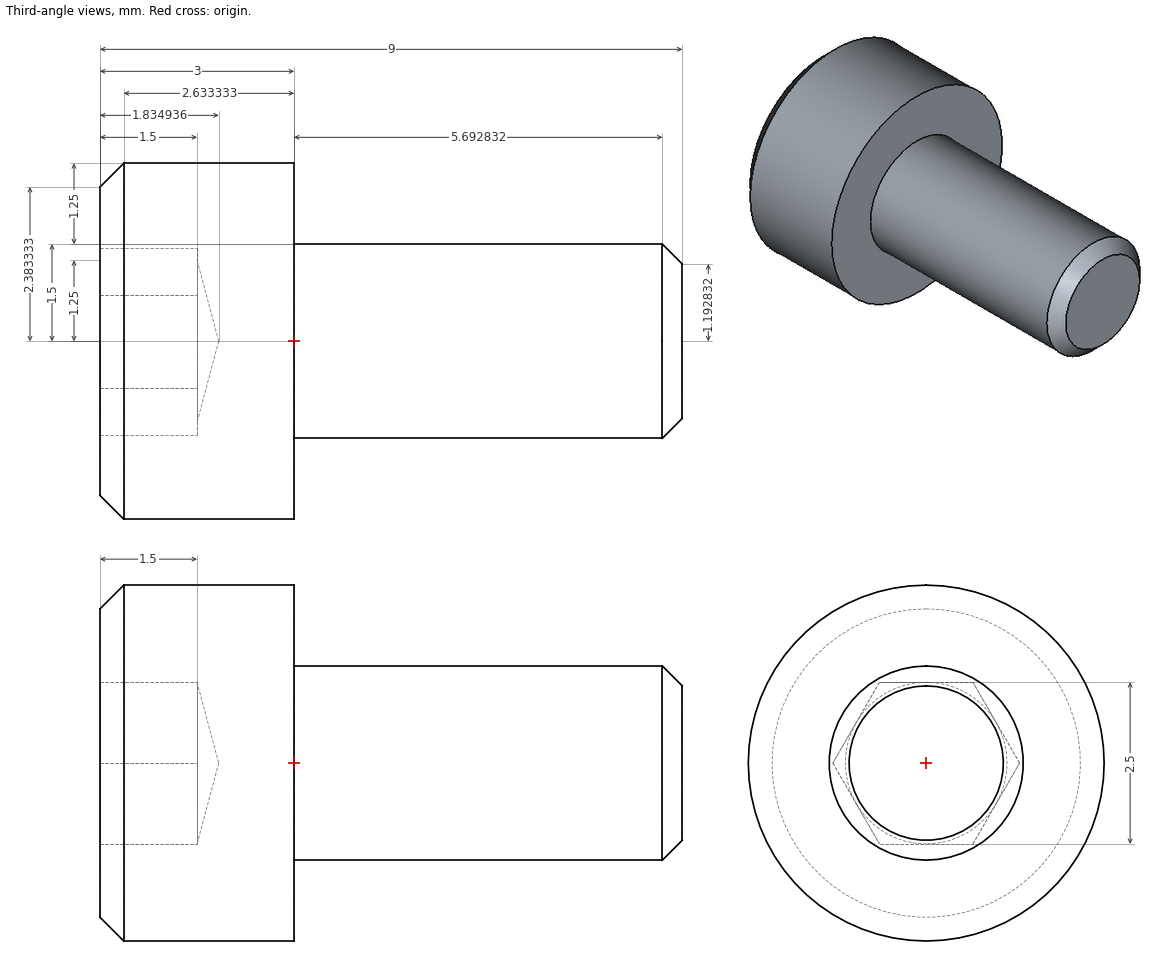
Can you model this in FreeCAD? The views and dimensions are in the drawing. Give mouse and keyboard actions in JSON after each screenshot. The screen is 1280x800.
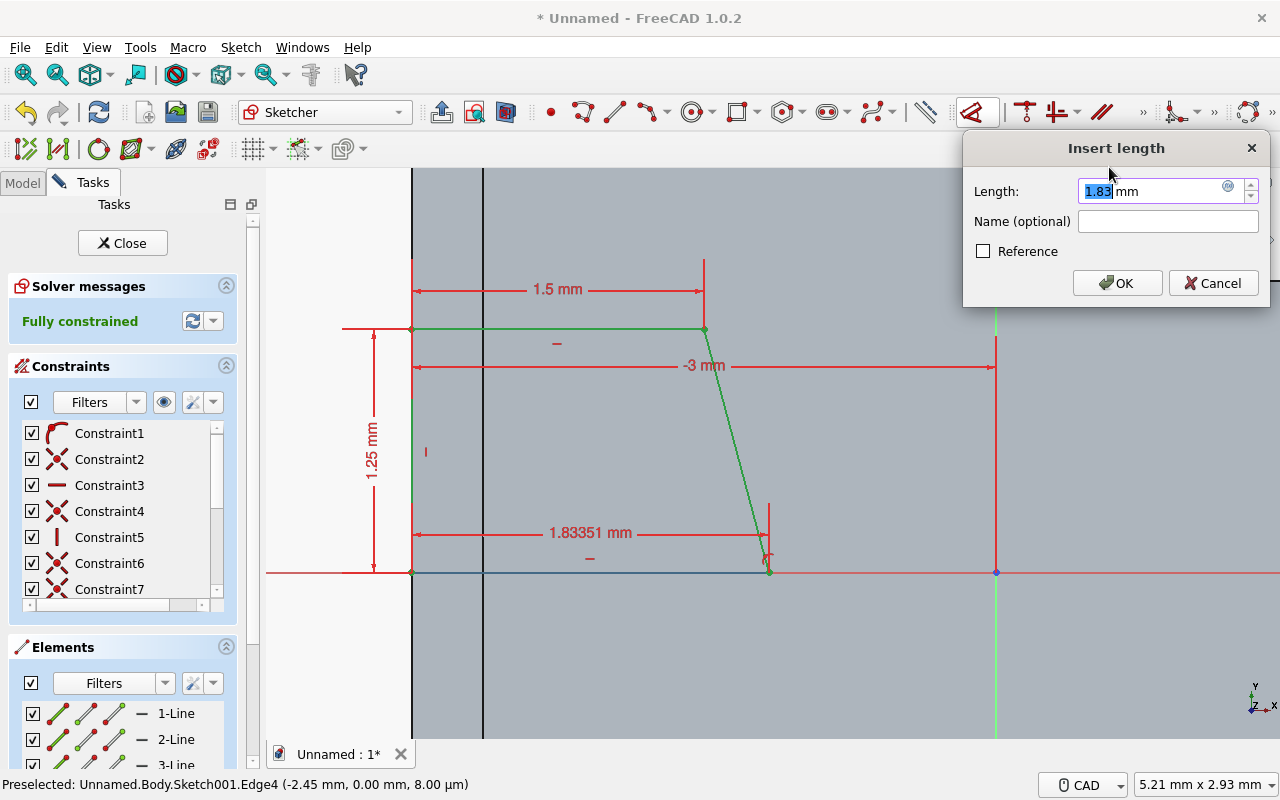
{"action": "type", "text": "1.834936"}
{"action": "key", "text": "Return"}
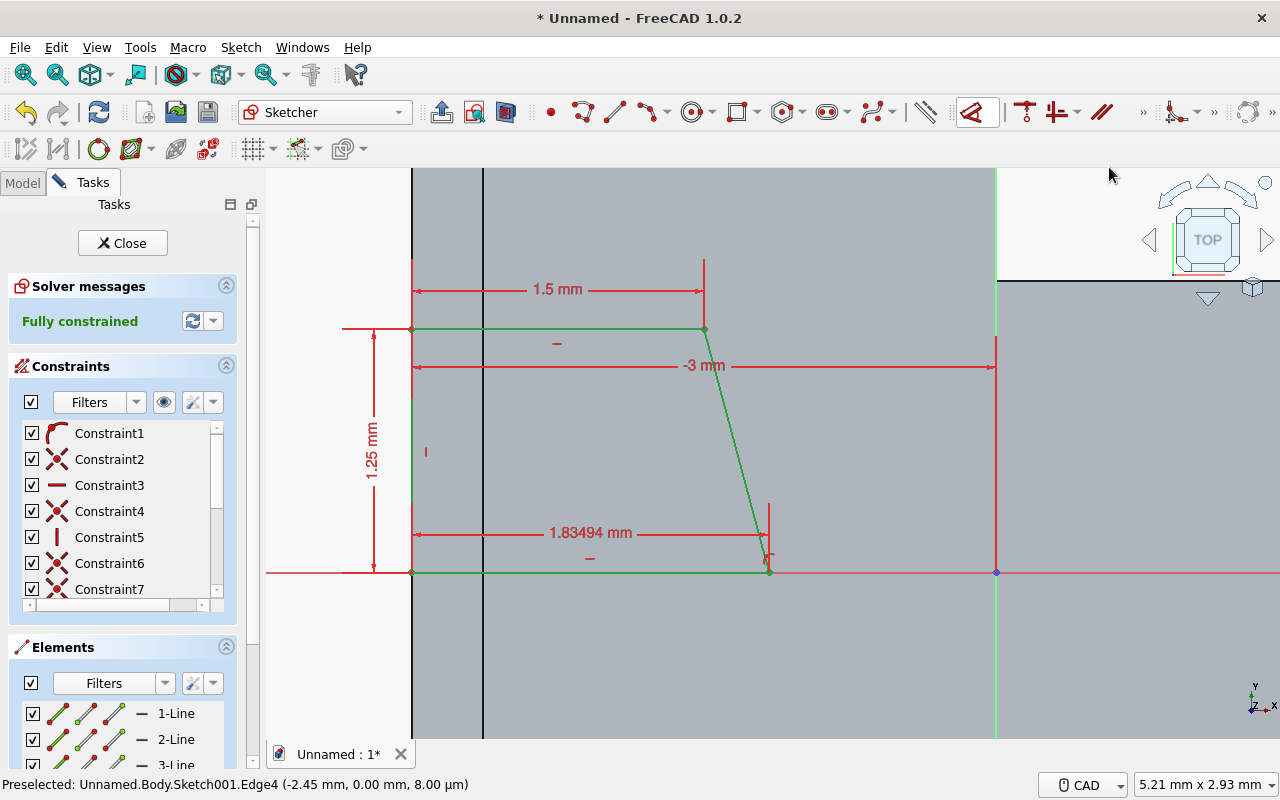
{"action": "left_click", "coordinate": [123, 243]}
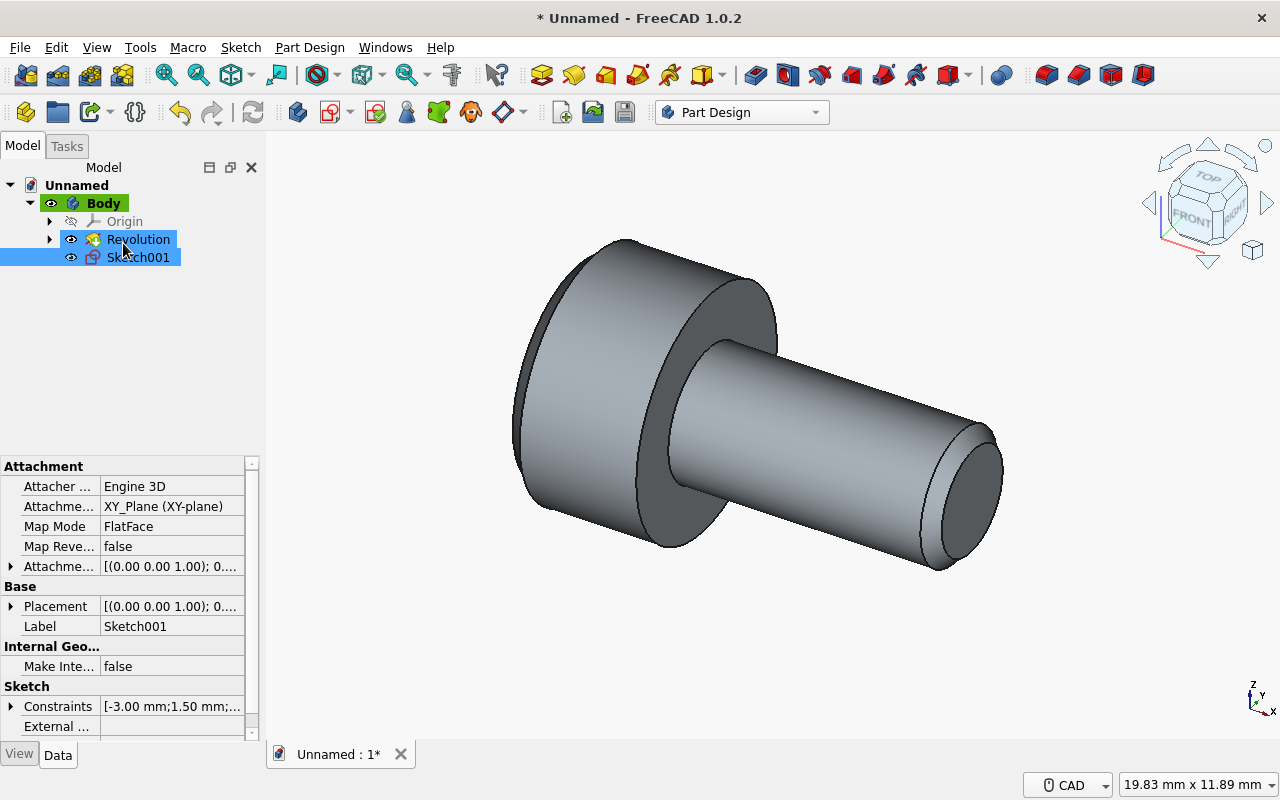
{"action": "left_click", "coordinate": [820, 76]}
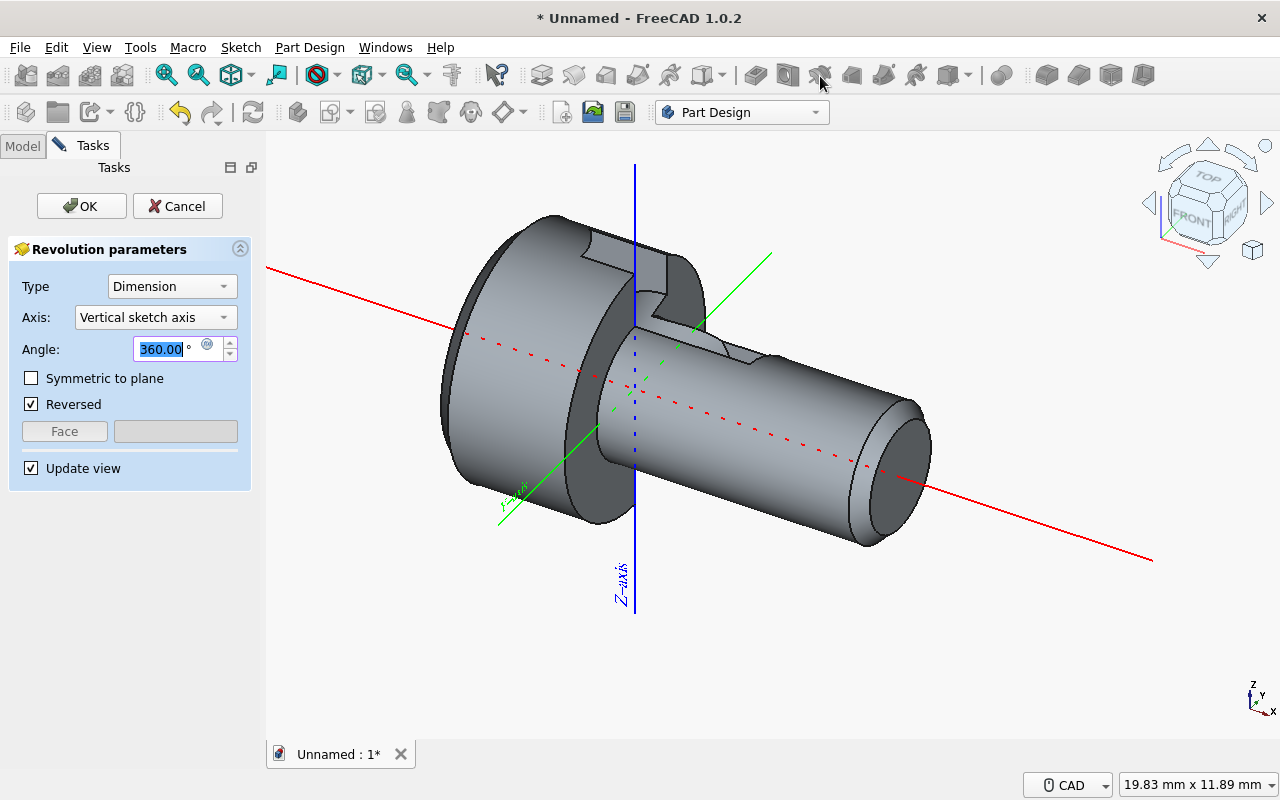
{"action": "left_click", "coordinate": [156, 318]}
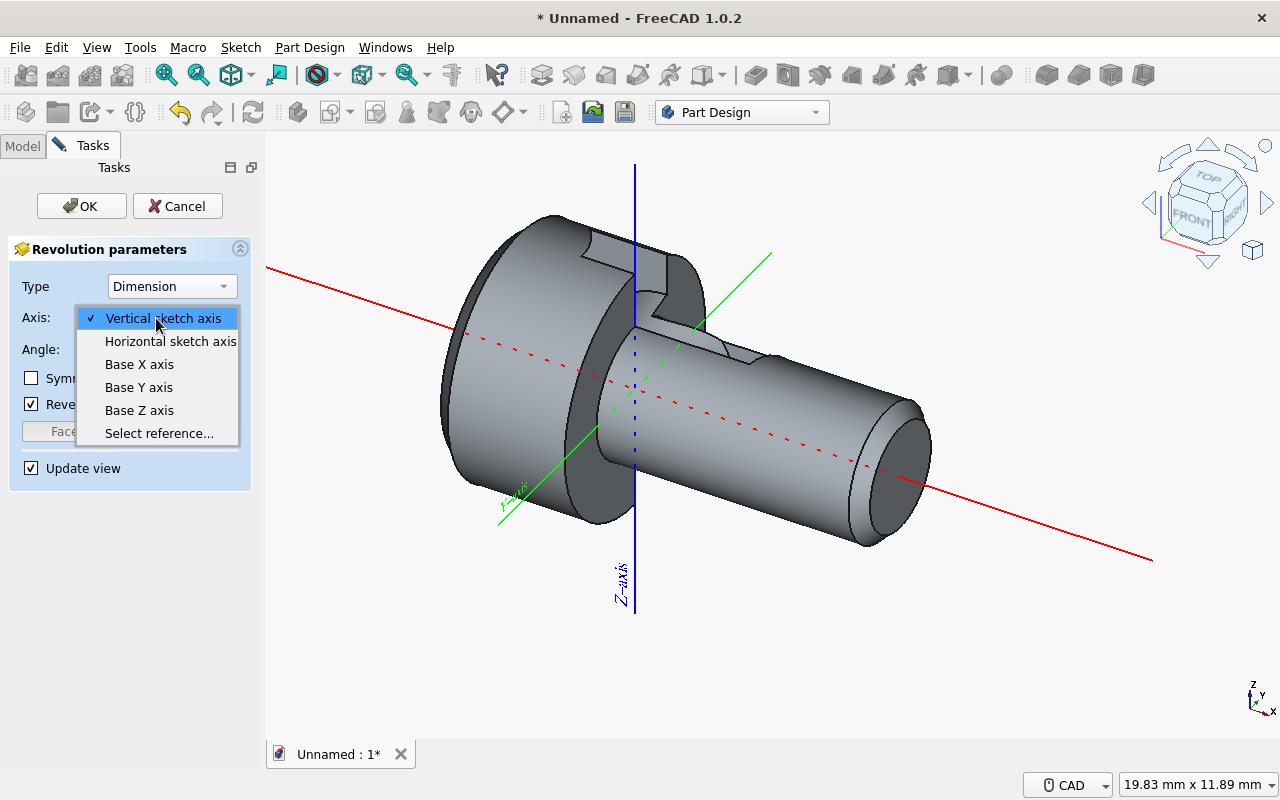
{"action": "left_click", "coordinate": [156, 342]}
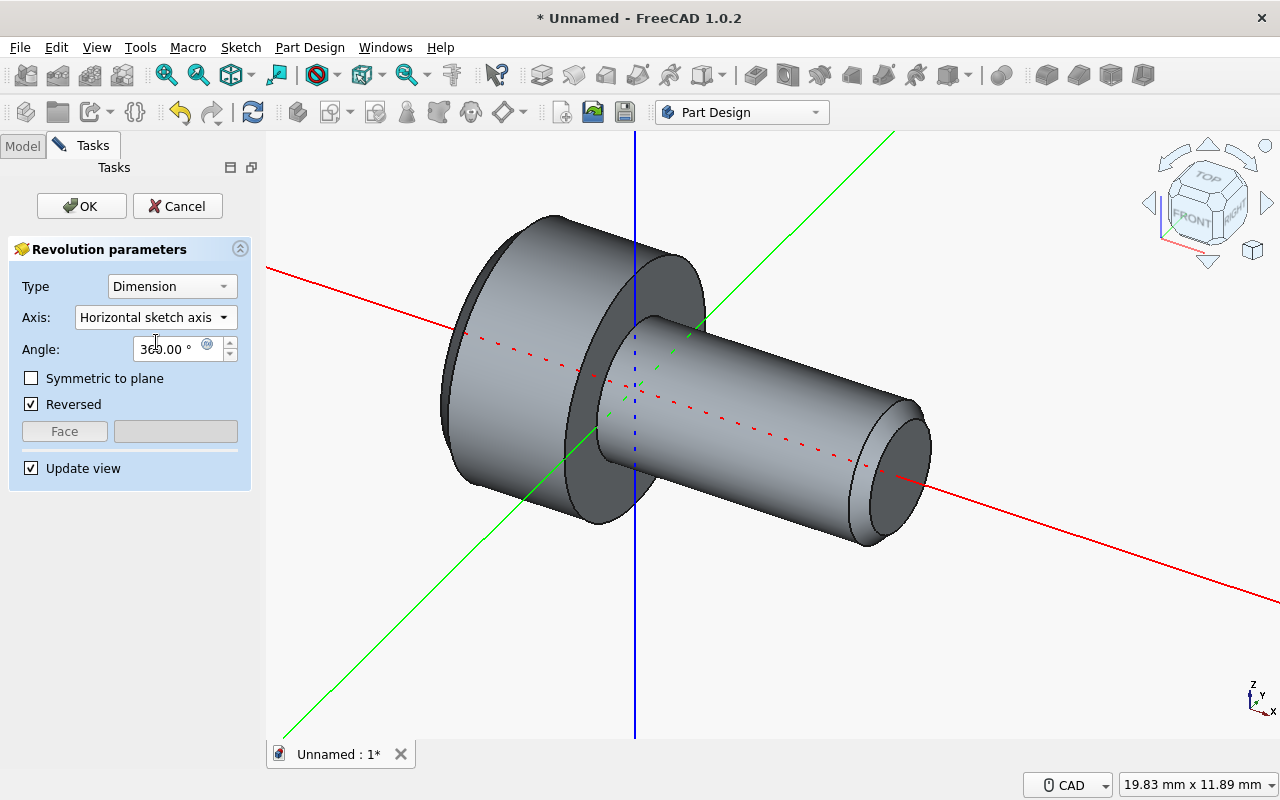
{"action": "left_click", "coordinate": [82, 206]}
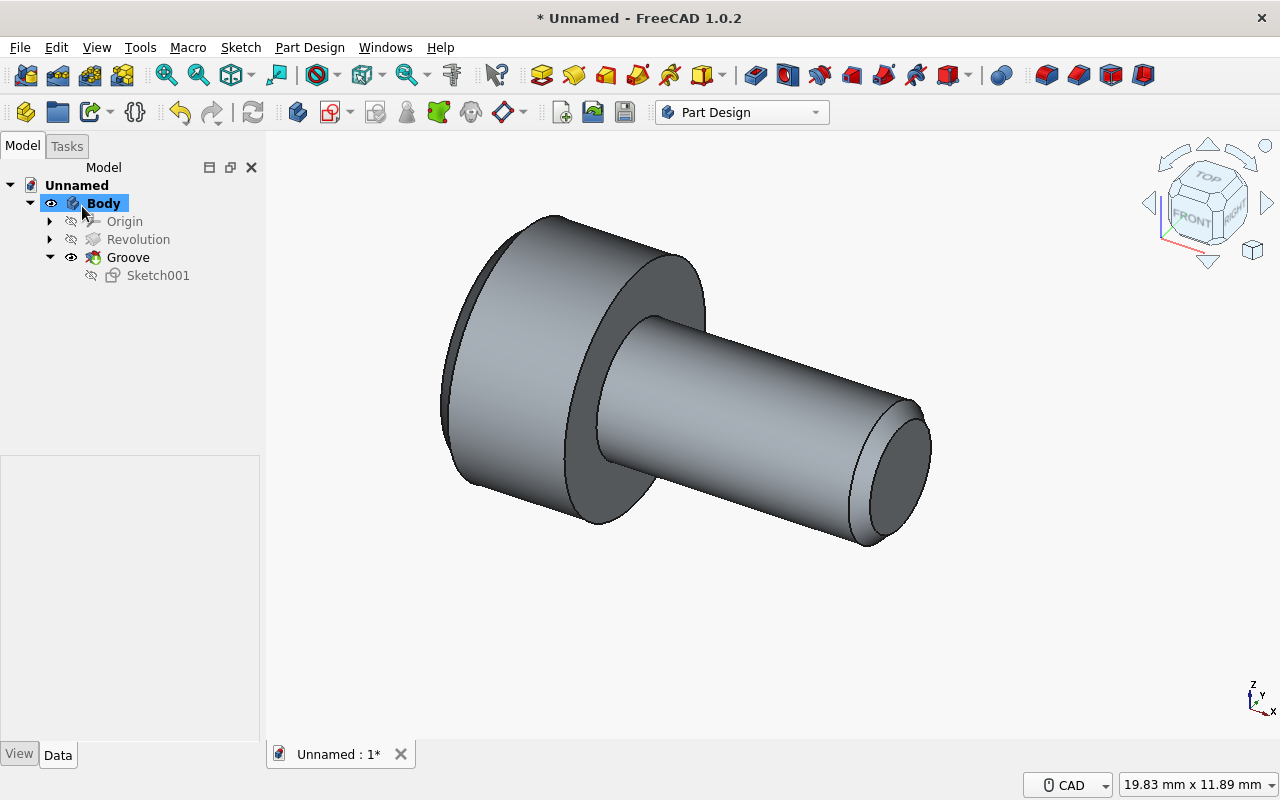
{"action": "key", "text": "6"}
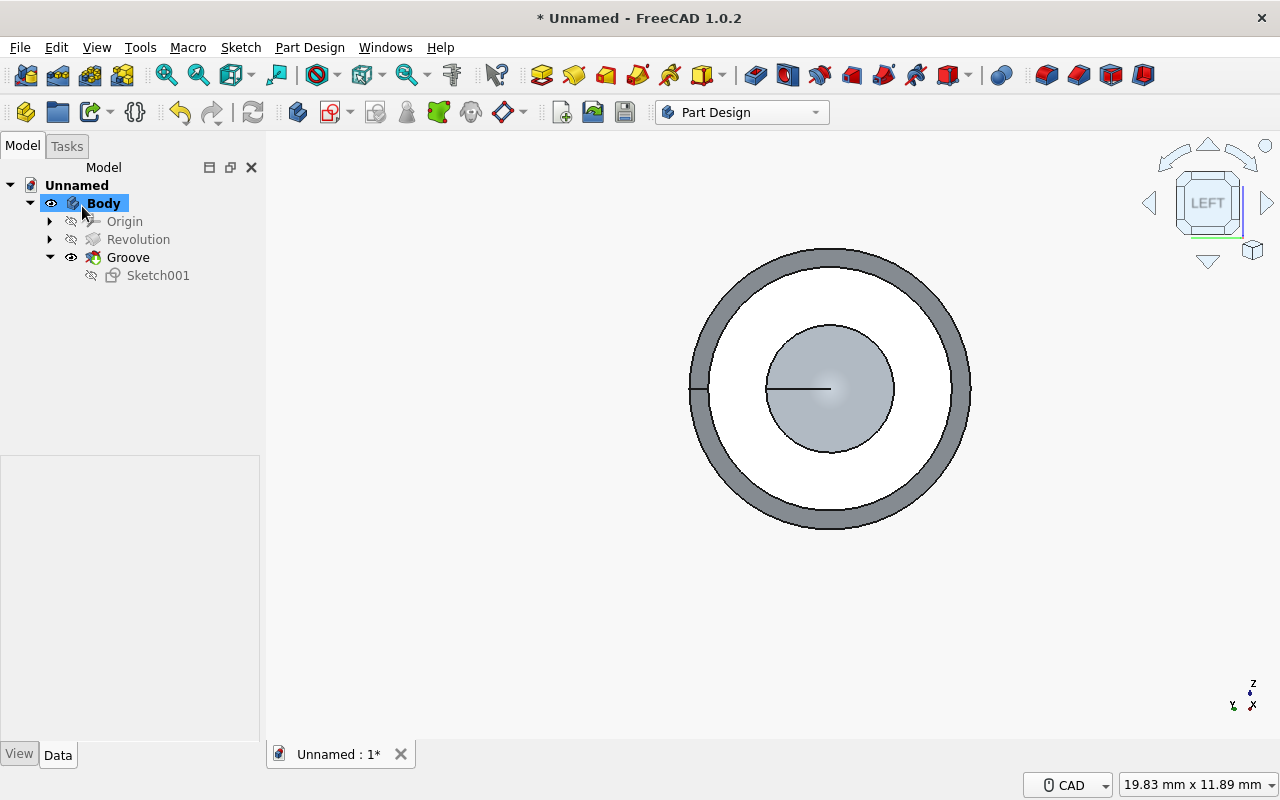
{"action": "left_click", "coordinate": [900, 458]}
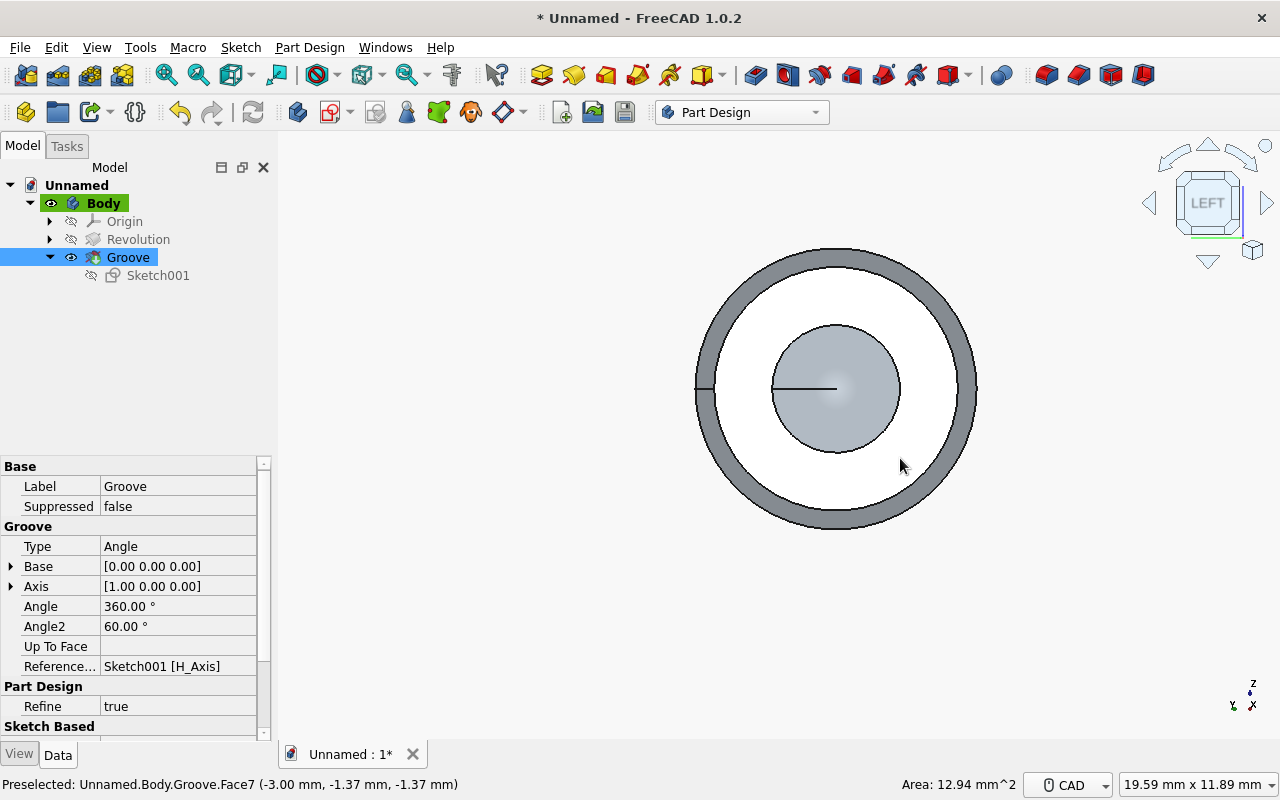
{"action": "left_click", "coordinate": [330, 112]}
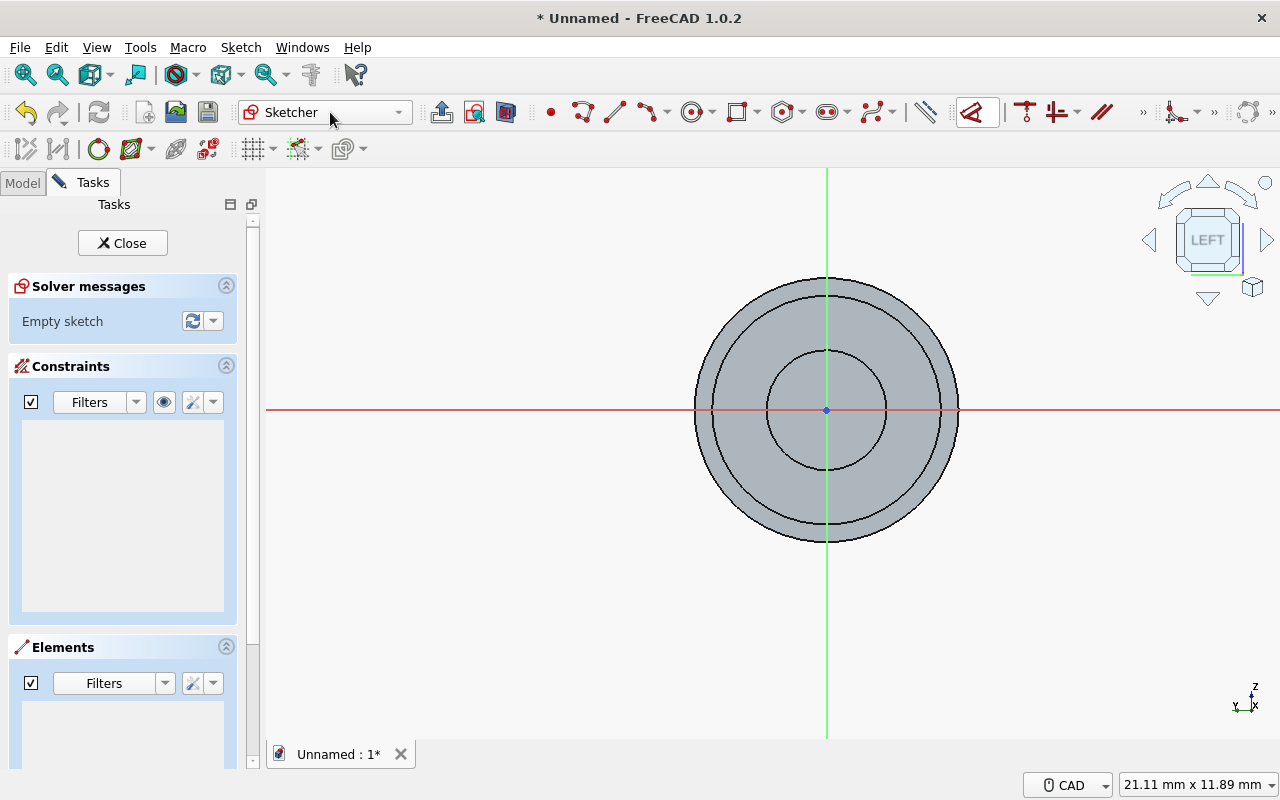
{"action": "scroll", "coordinate": [879, 392], "scroll_direction": "up", "scroll_amount": 6}